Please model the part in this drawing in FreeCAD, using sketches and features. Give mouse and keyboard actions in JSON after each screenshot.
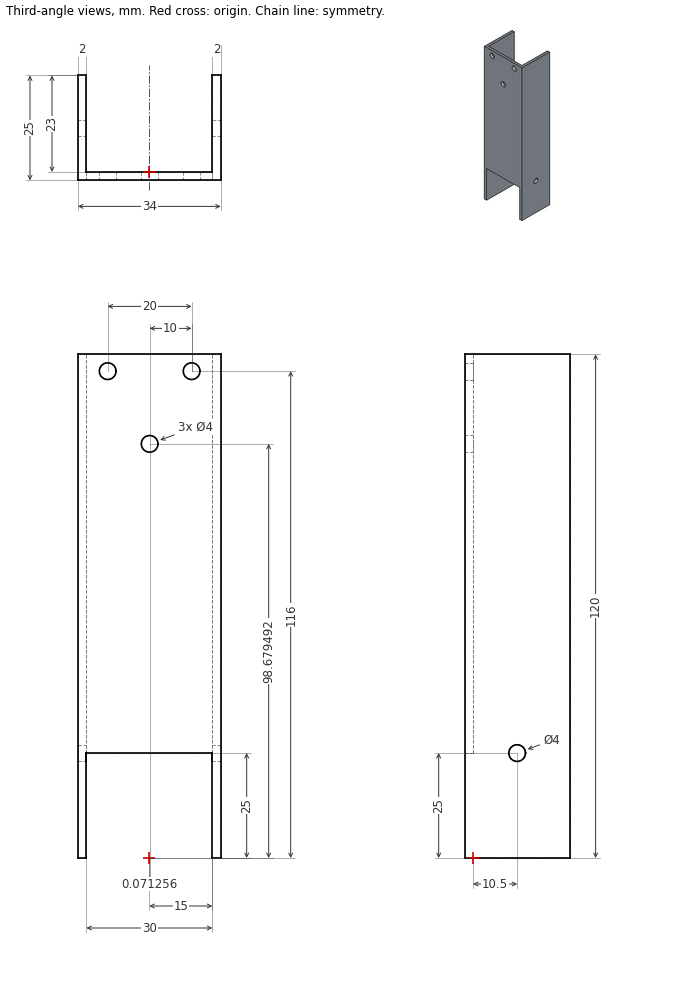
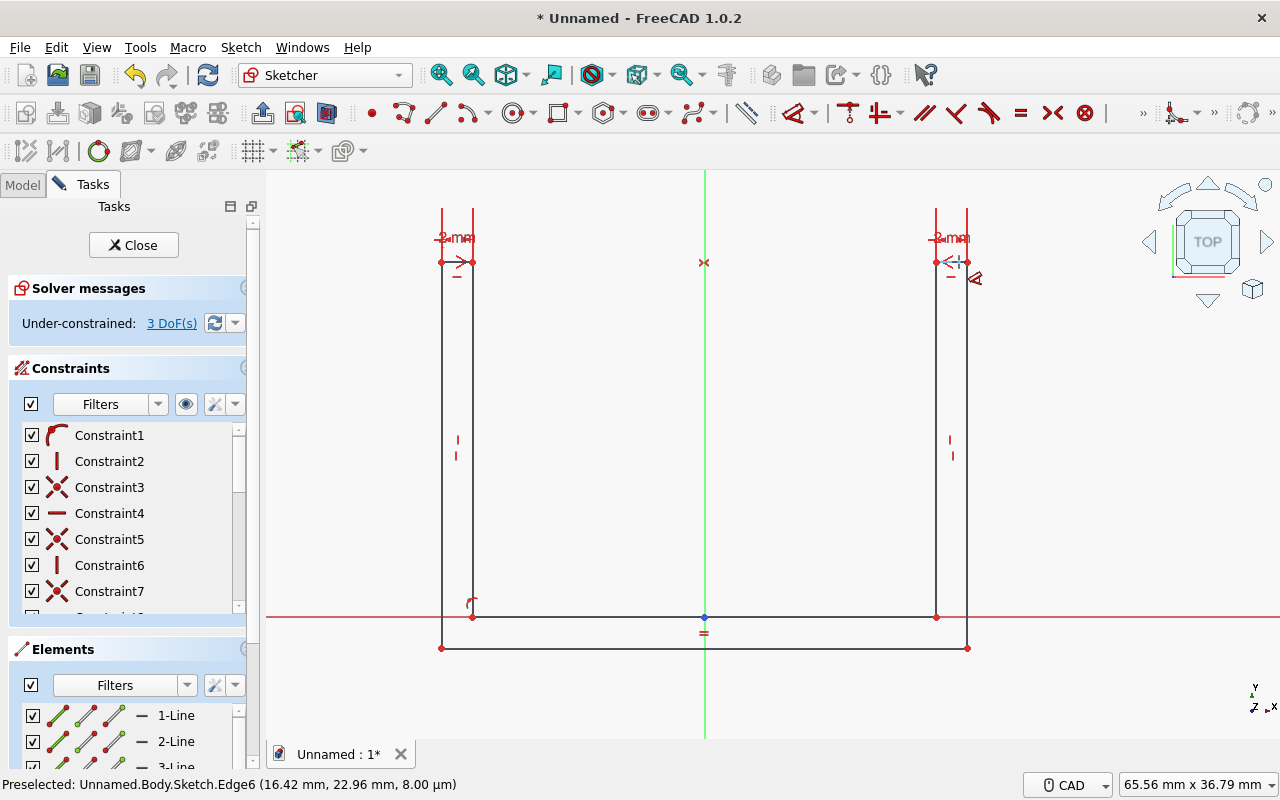
{"action": "left_click", "coordinate": [473, 511]}
{"action": "left_click", "coordinate": [507, 440]}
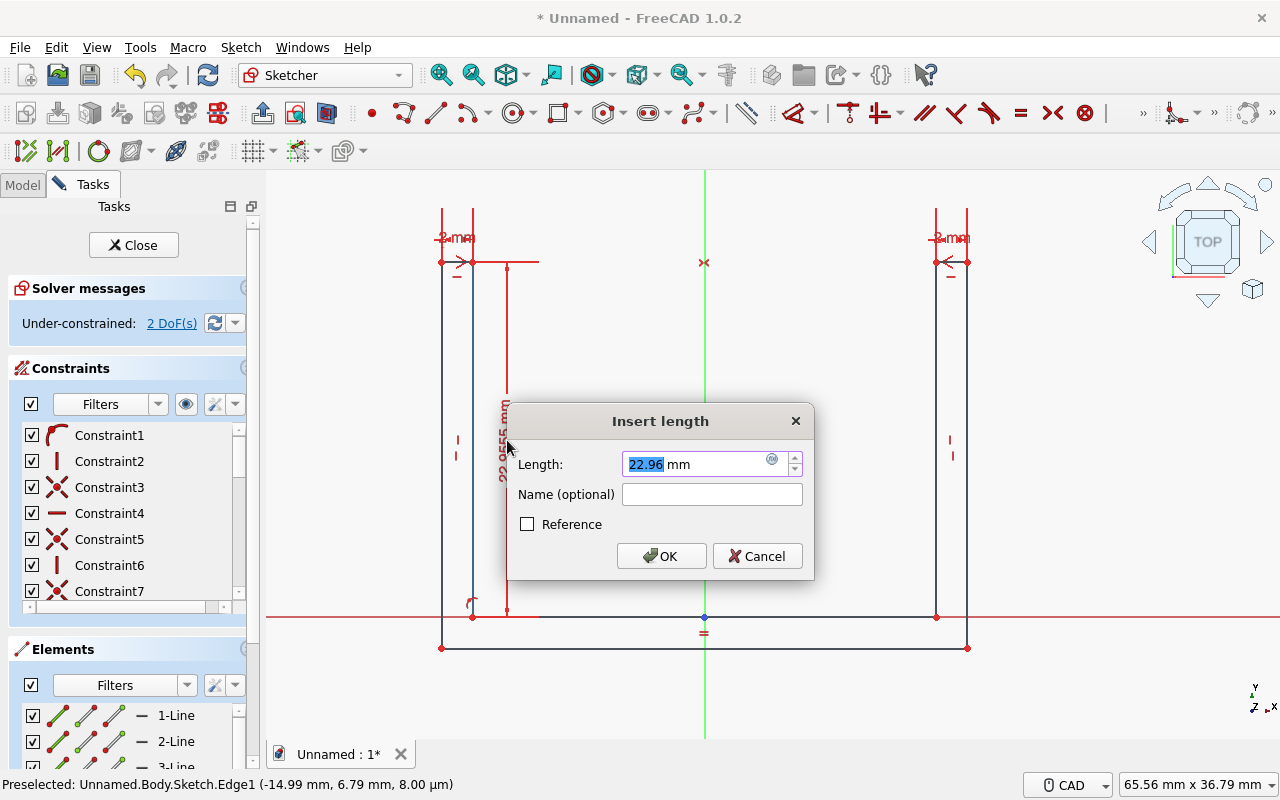
{"action": "type", "text": "23"}
{"action": "key", "text": "Return"}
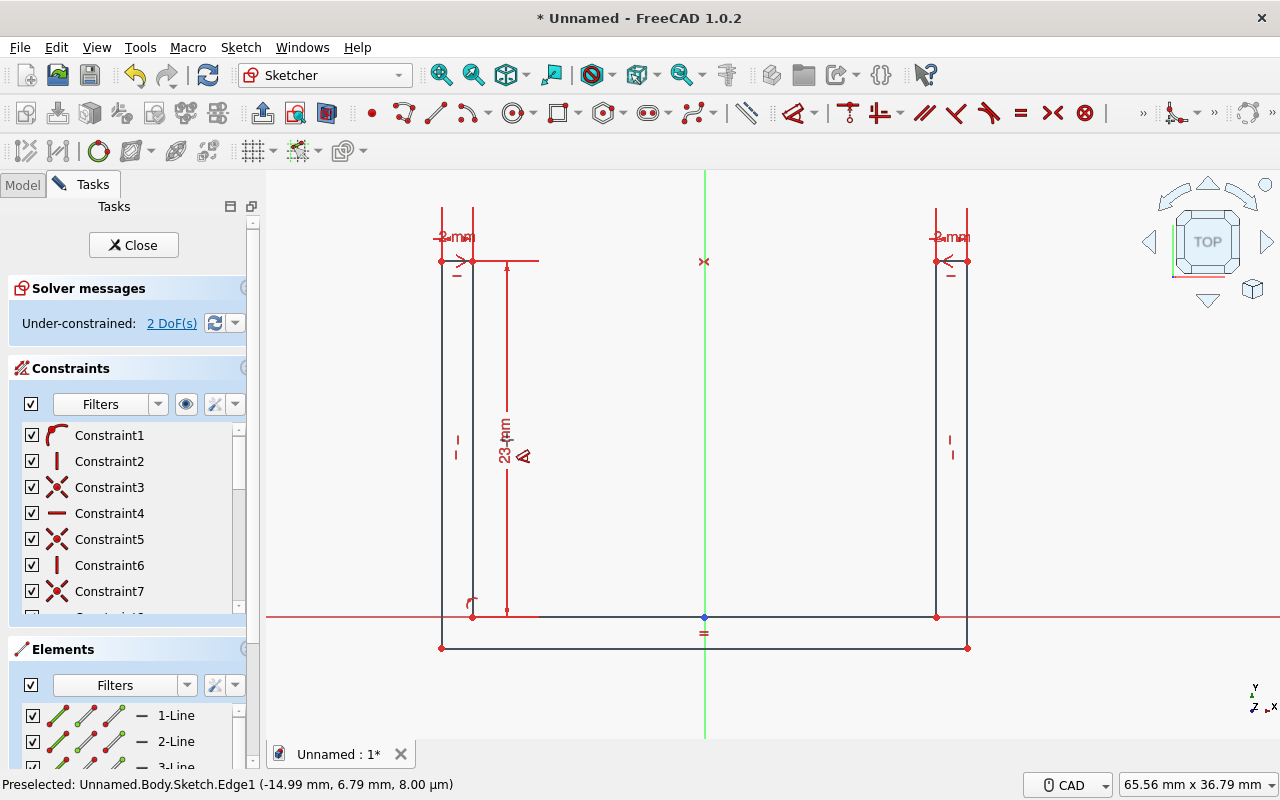
{"action": "left_click", "coordinate": [442, 378]}
{"action": "left_click", "coordinate": [408, 455]}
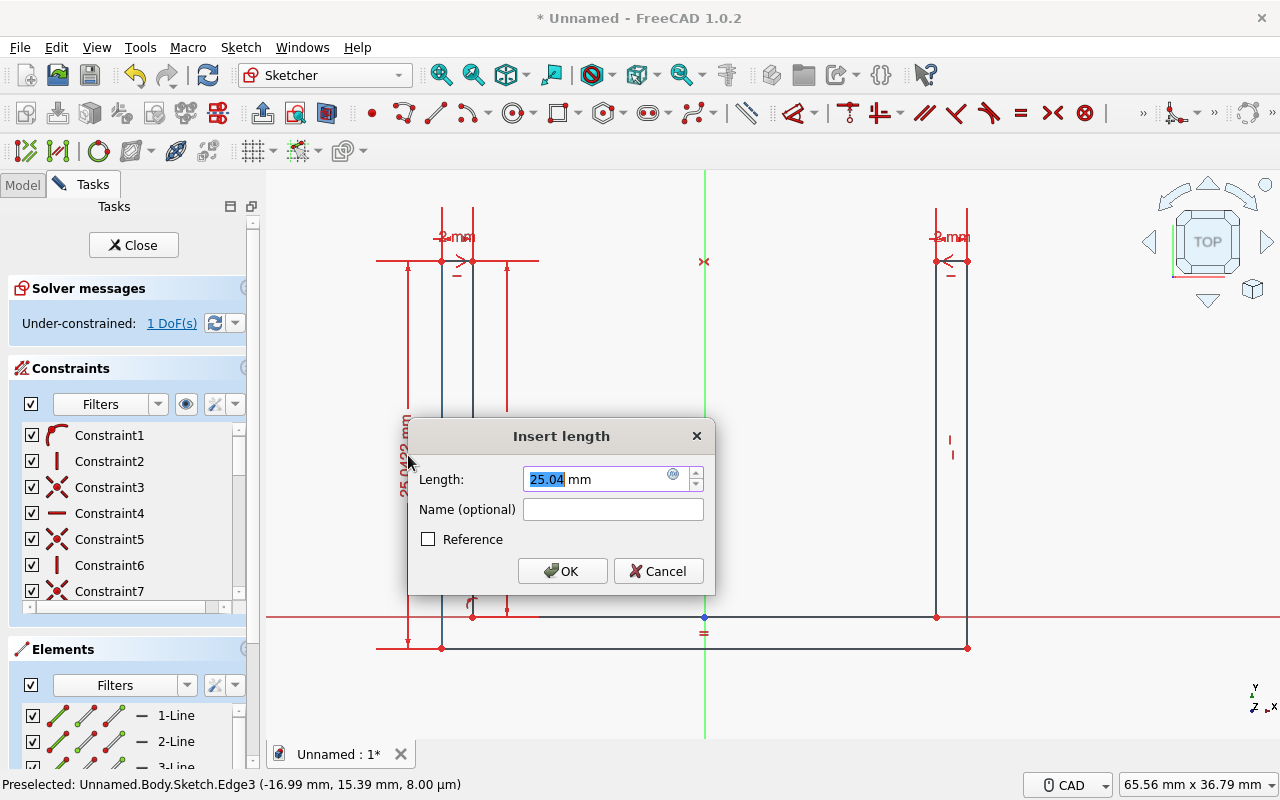
{"action": "type", "text": "25"}
{"action": "key", "text": "Return"}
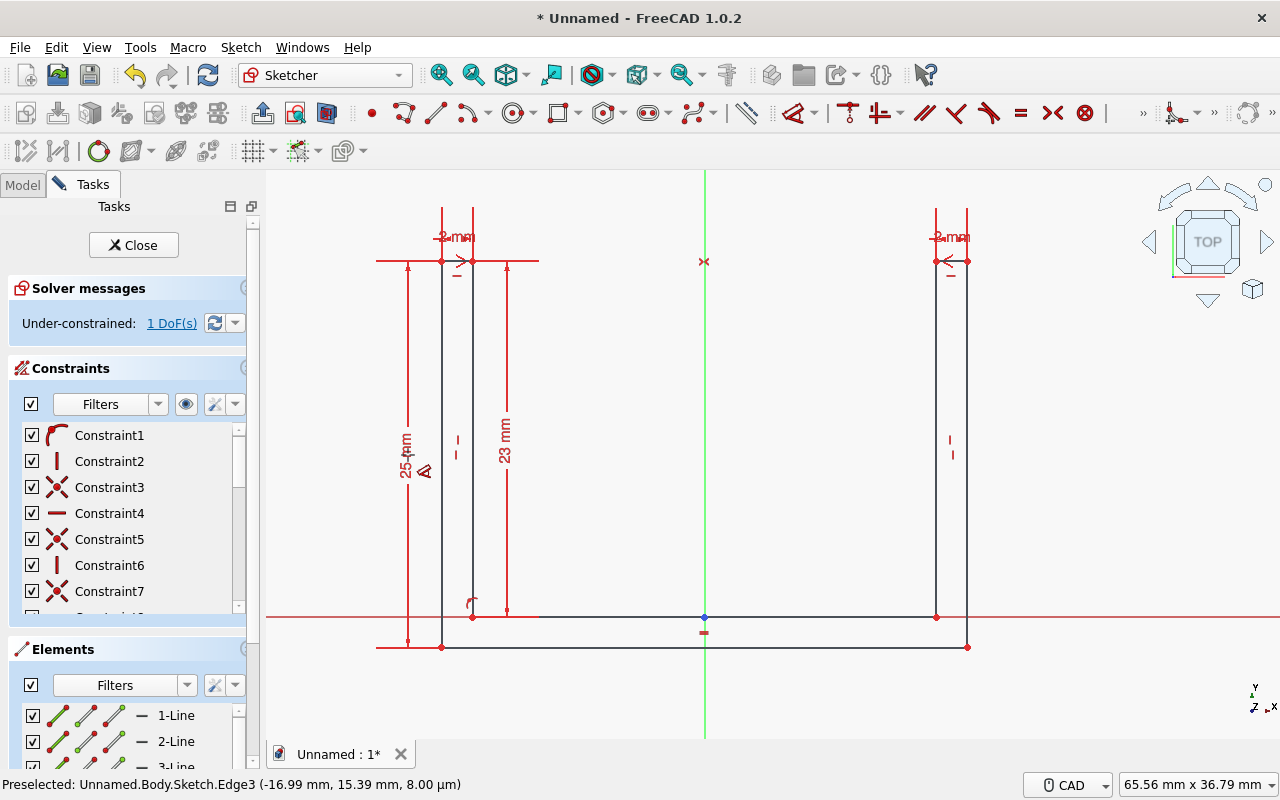
{"action": "left_click", "coordinate": [599, 648]}
{"action": "left_click", "coordinate": [584, 682]}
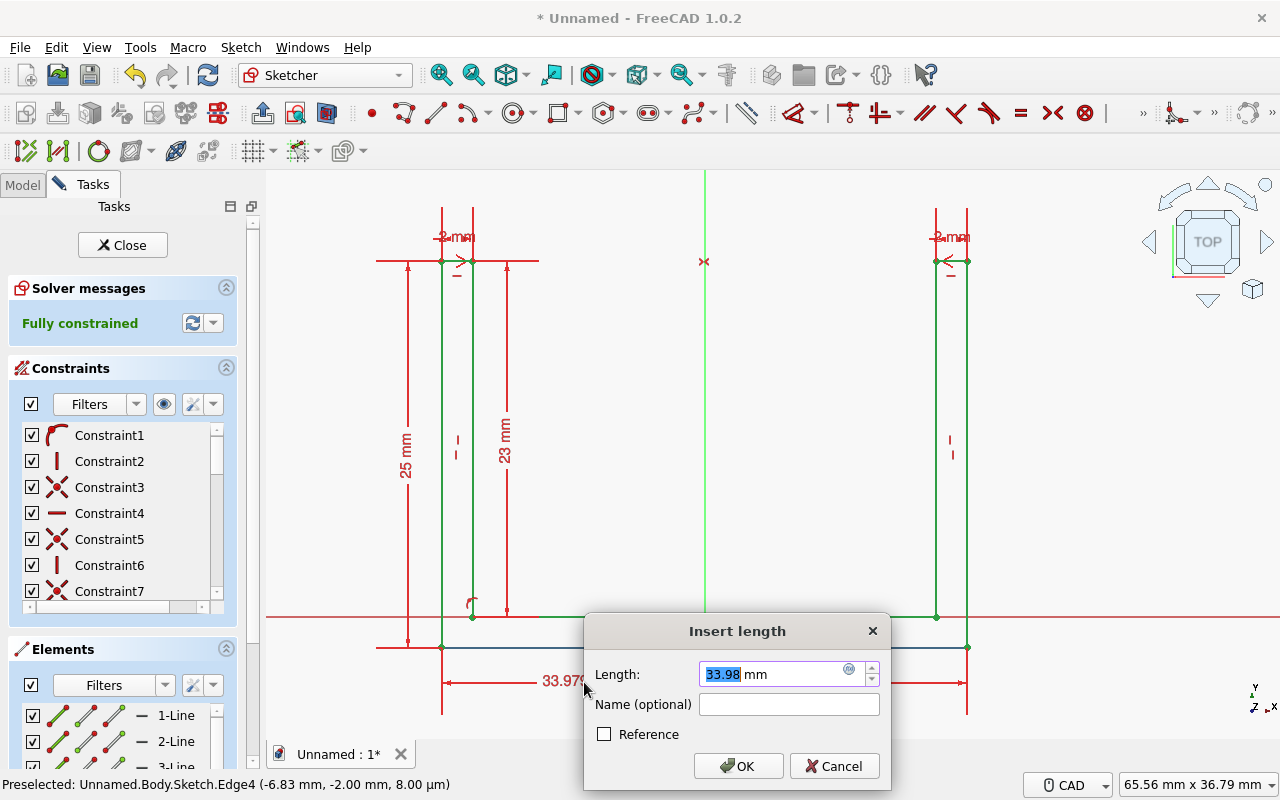
{"action": "type", "text": "34"}
{"action": "key", "text": "Return"}
{"action": "key", "text": "Escape"}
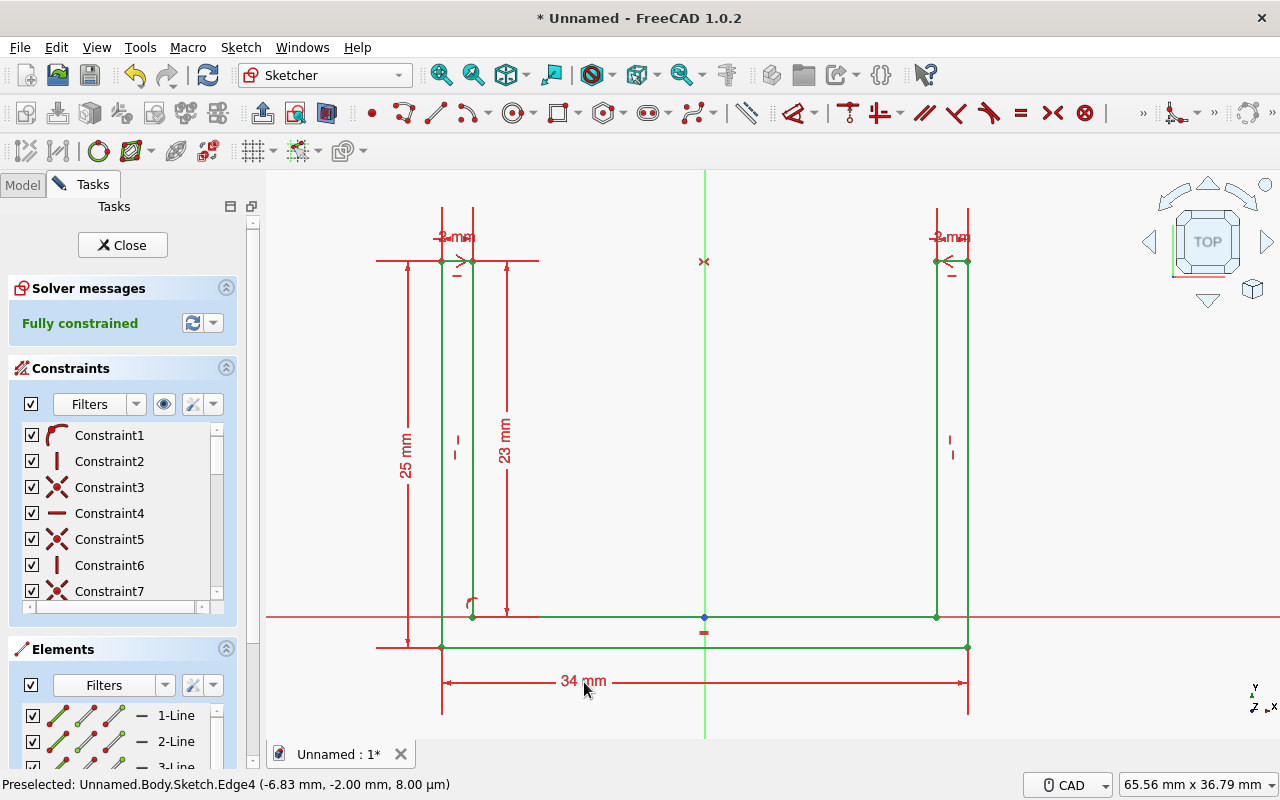
{"action": "left_click", "coordinate": [123, 245]}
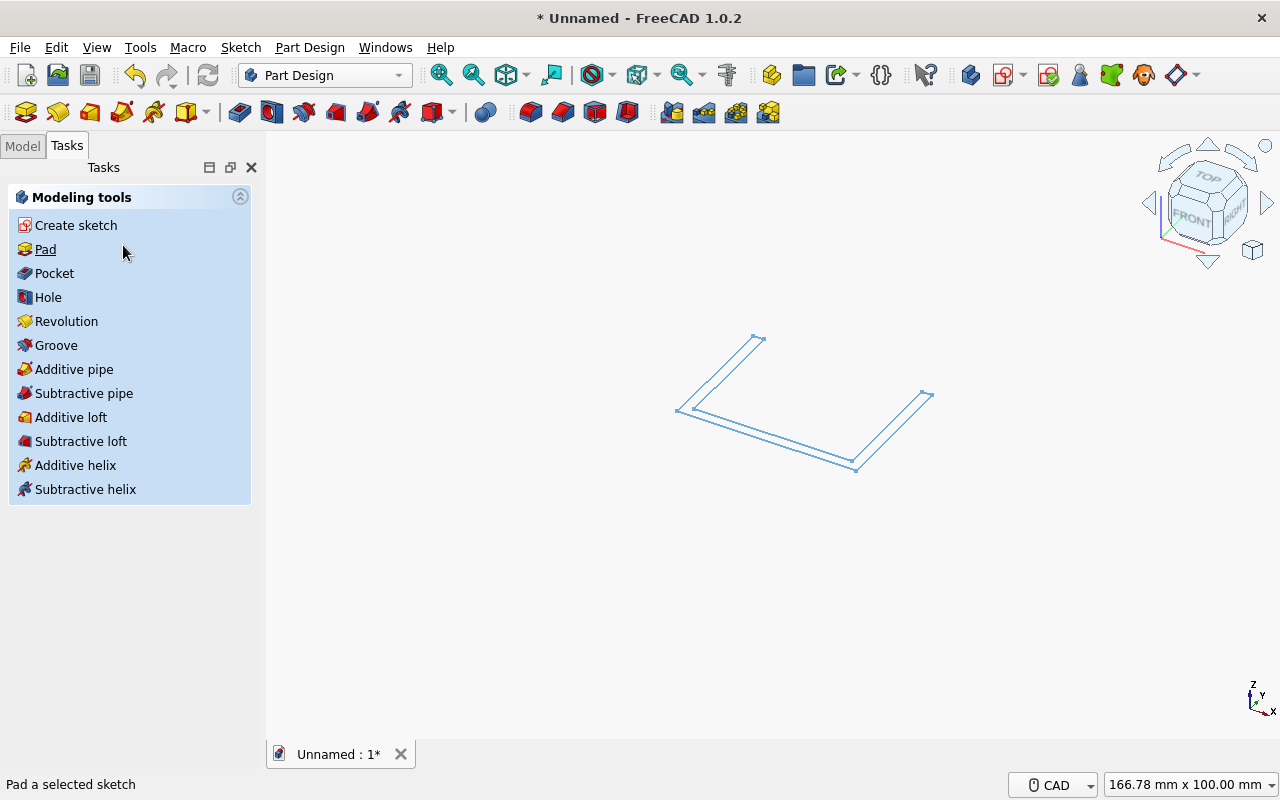
{"action": "left_click", "coordinate": [26, 112]}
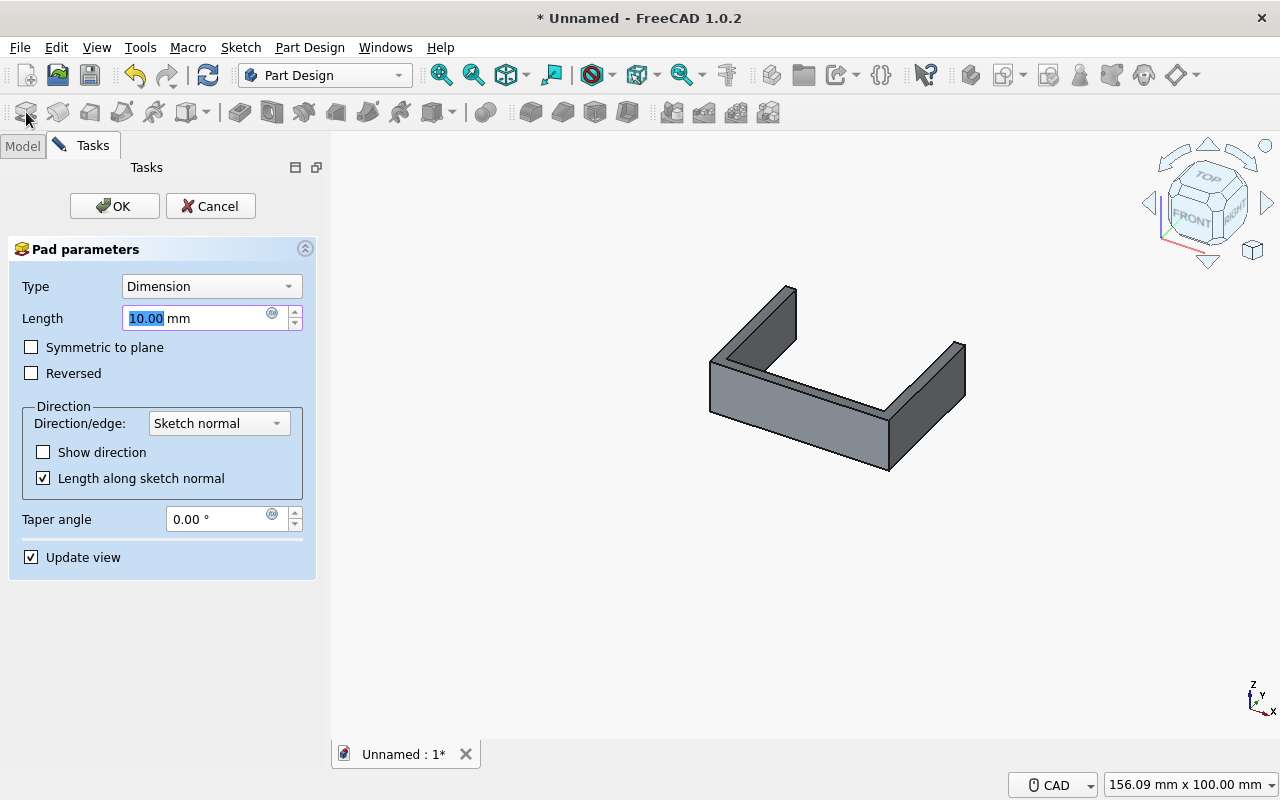
{"action": "type", "text": "120"}
{"action": "key", "text": "Tab"}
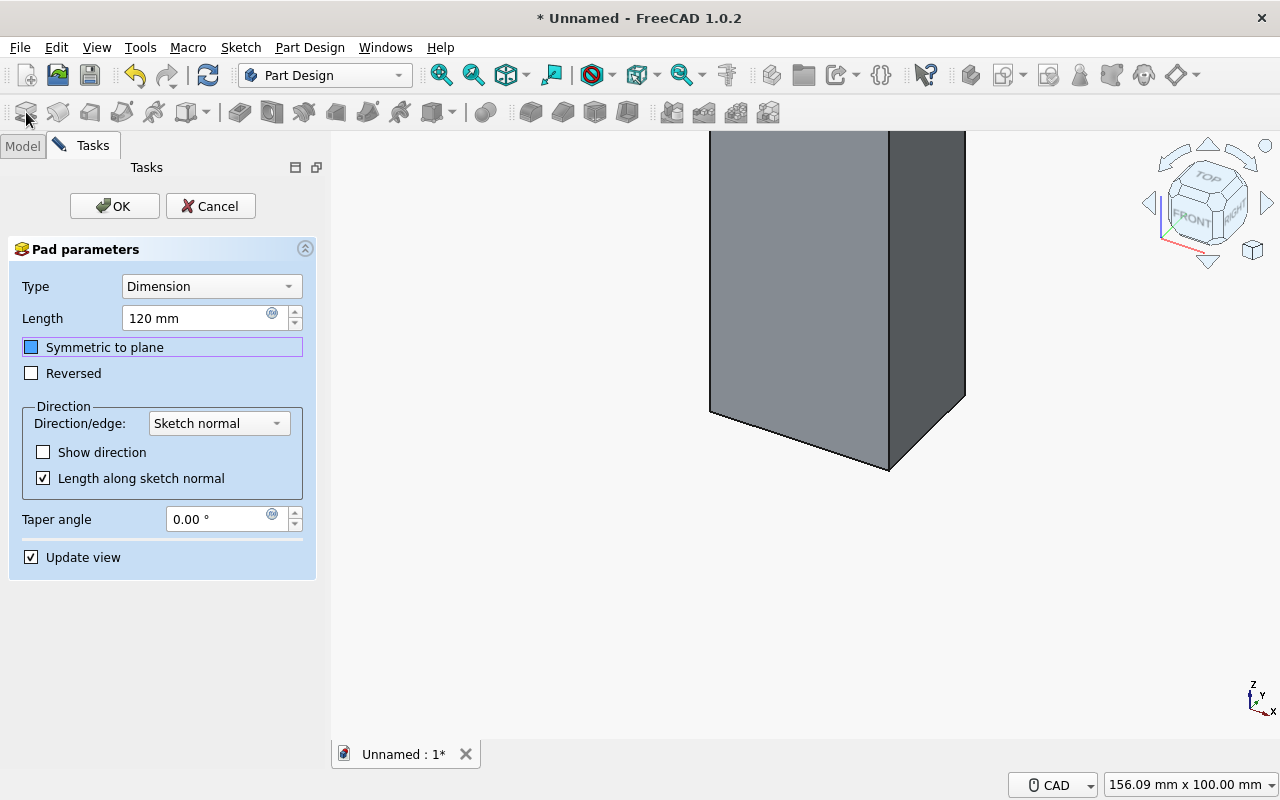
{"action": "left_click", "coordinate": [115, 206]}